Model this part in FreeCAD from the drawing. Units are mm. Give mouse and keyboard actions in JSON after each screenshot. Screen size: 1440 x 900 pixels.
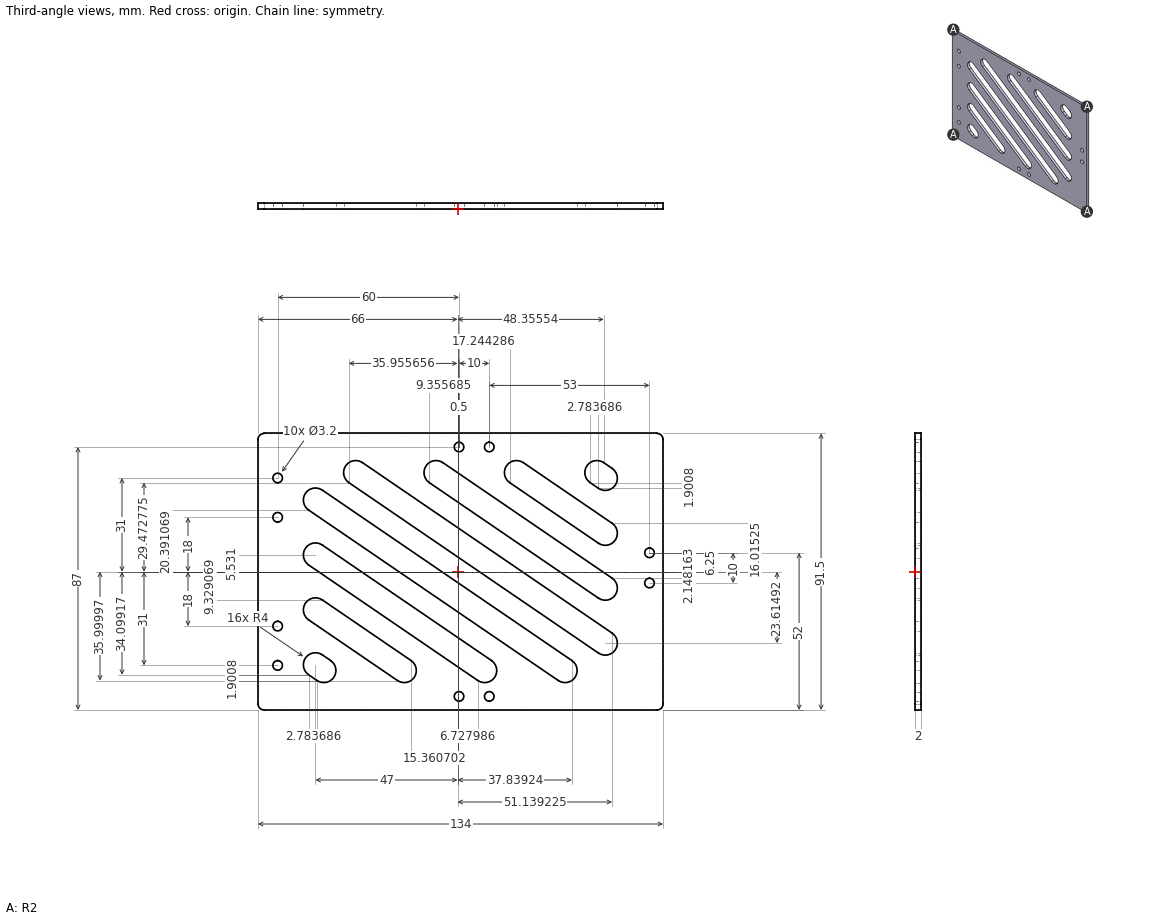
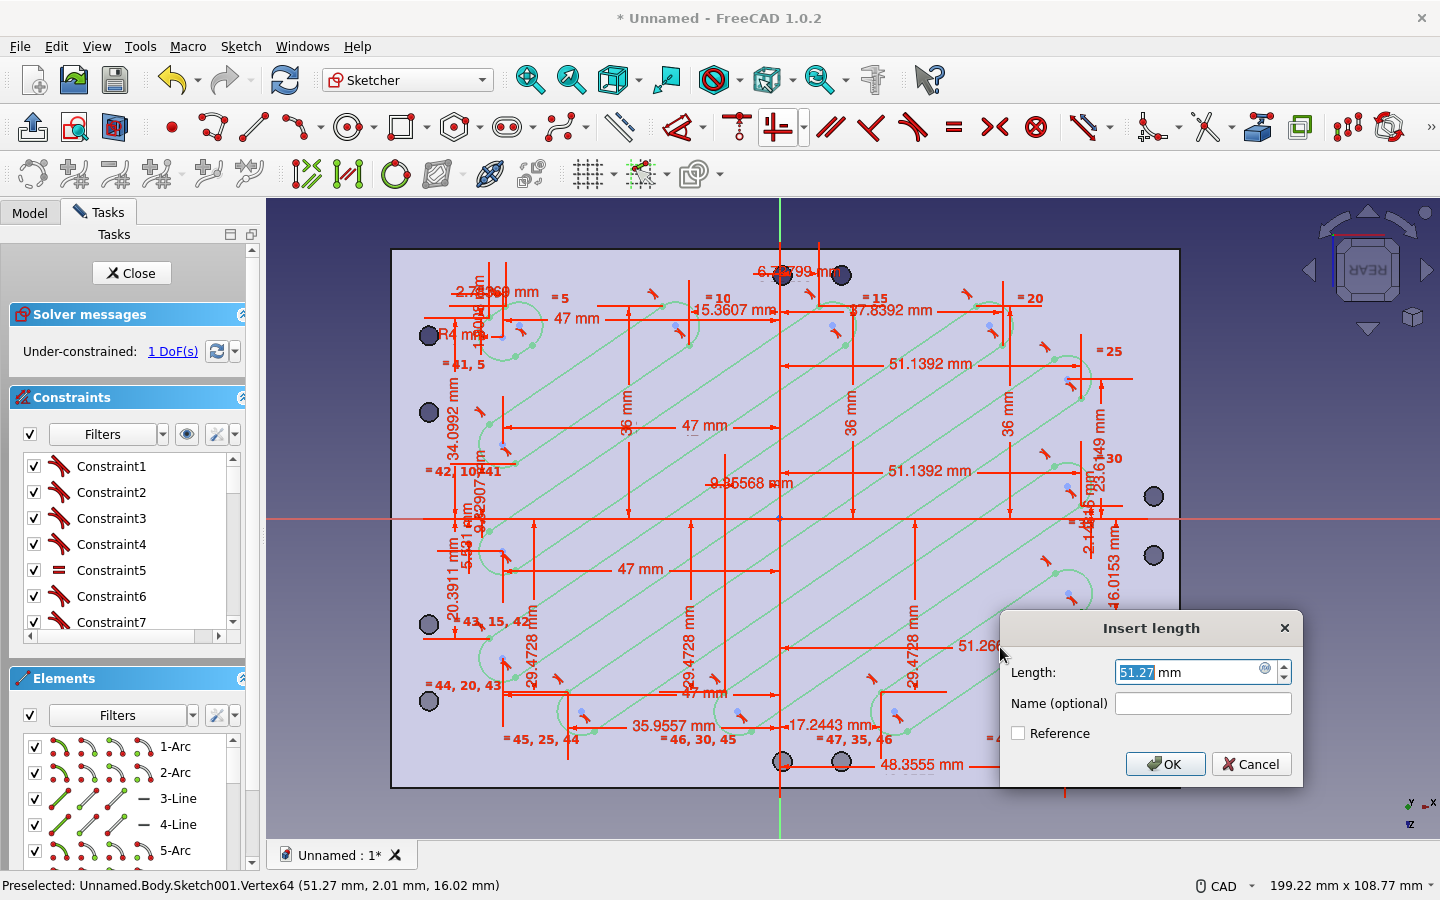
{"action": "type", "text": "51.139225"}
{"action": "key", "text": "Return"}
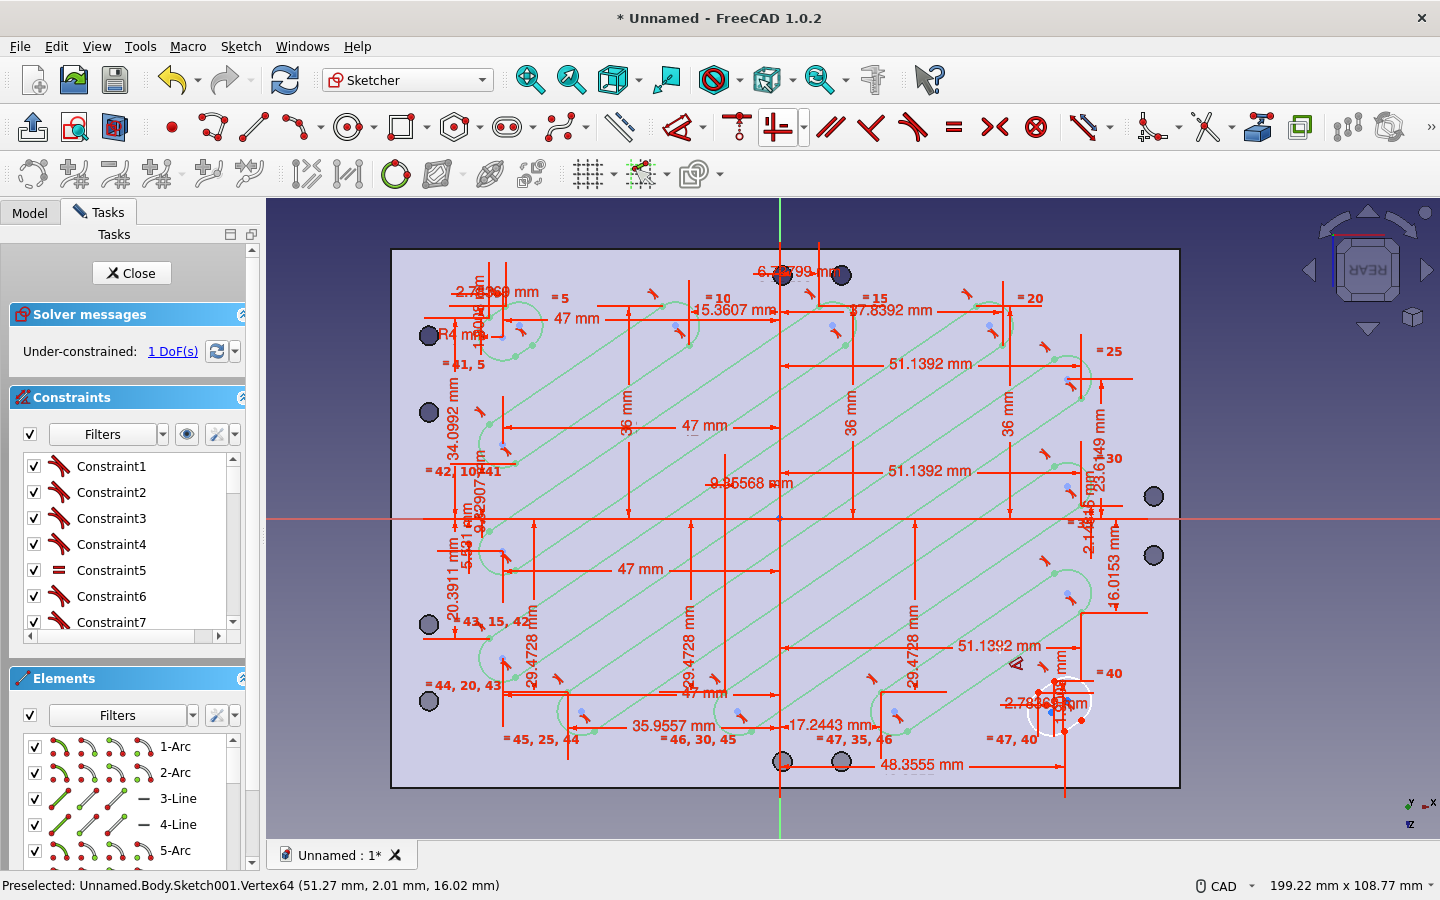
{"action": "left_click", "coordinate": [1038, 693]}
{"action": "left_click", "coordinate": [1072, 646]}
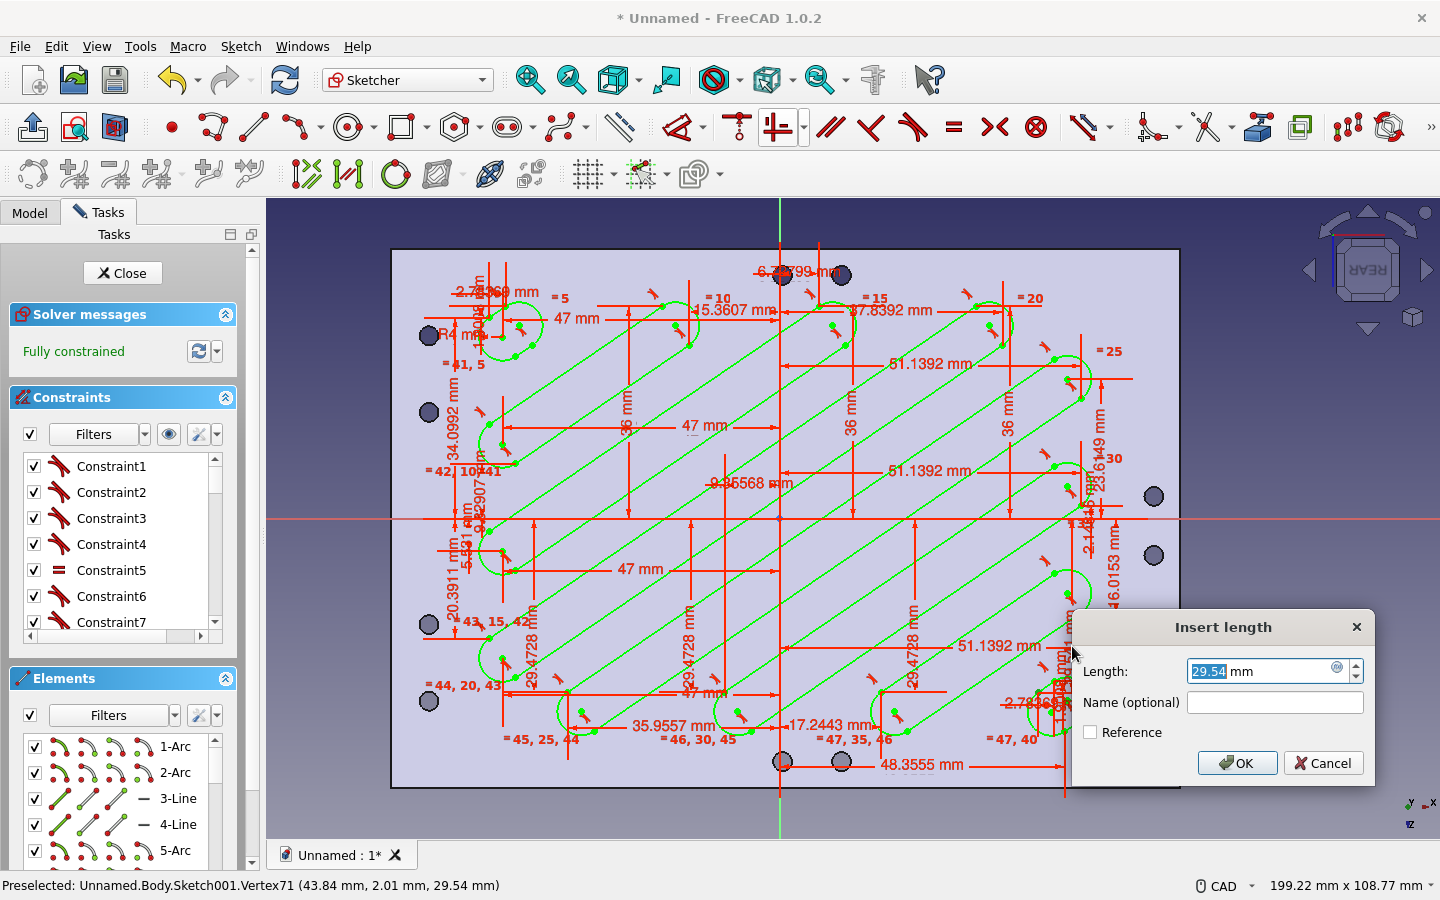
{"action": "type", "text": "29.472775"}
{"action": "key", "text": "Return"}
{"action": "key", "text": "Escape"}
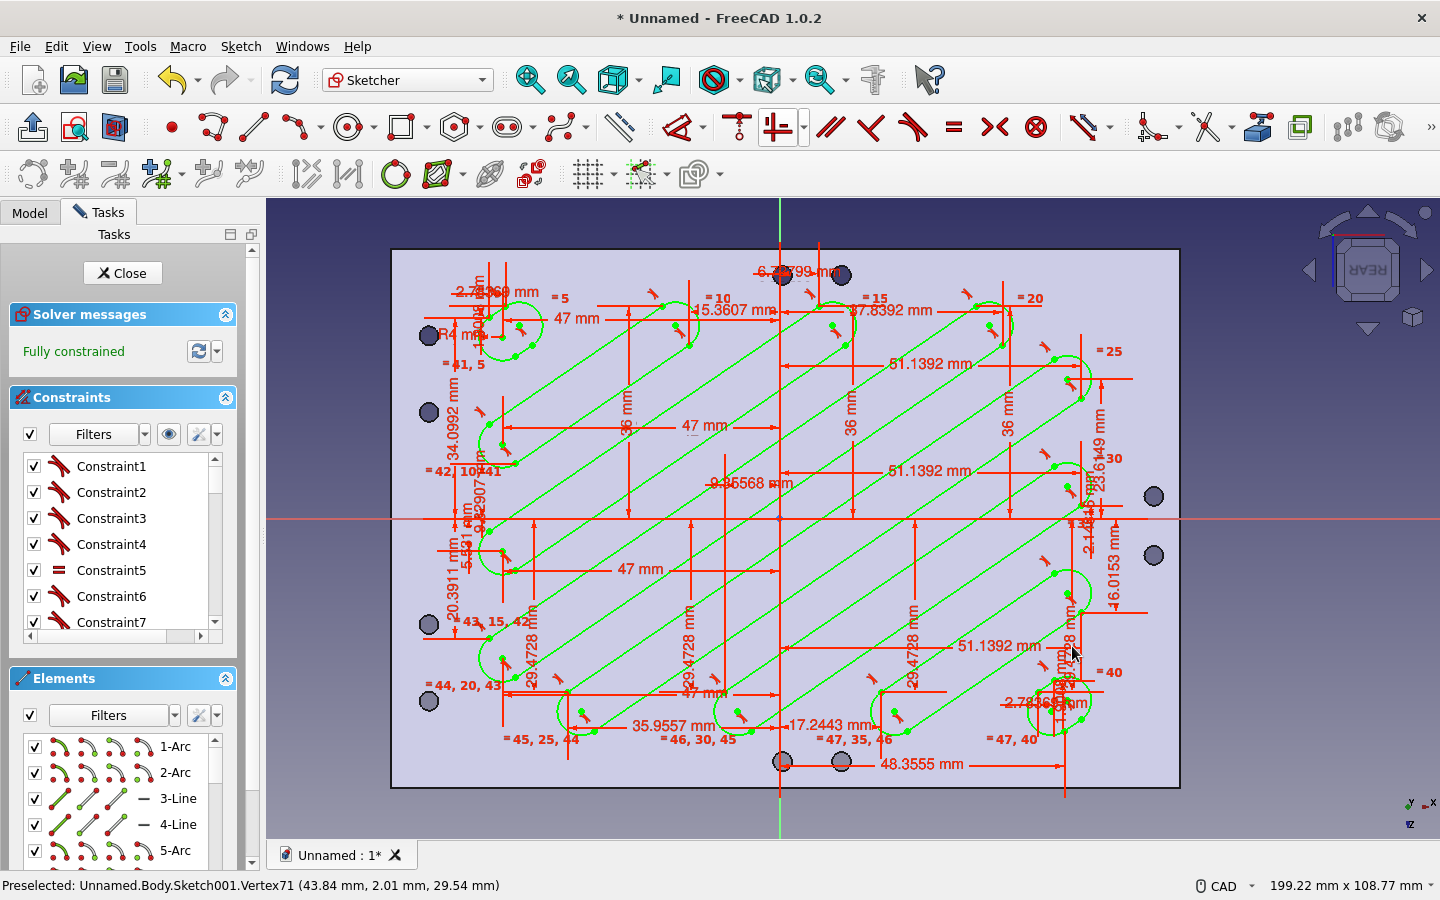
{"action": "left_click", "coordinate": [123, 273]}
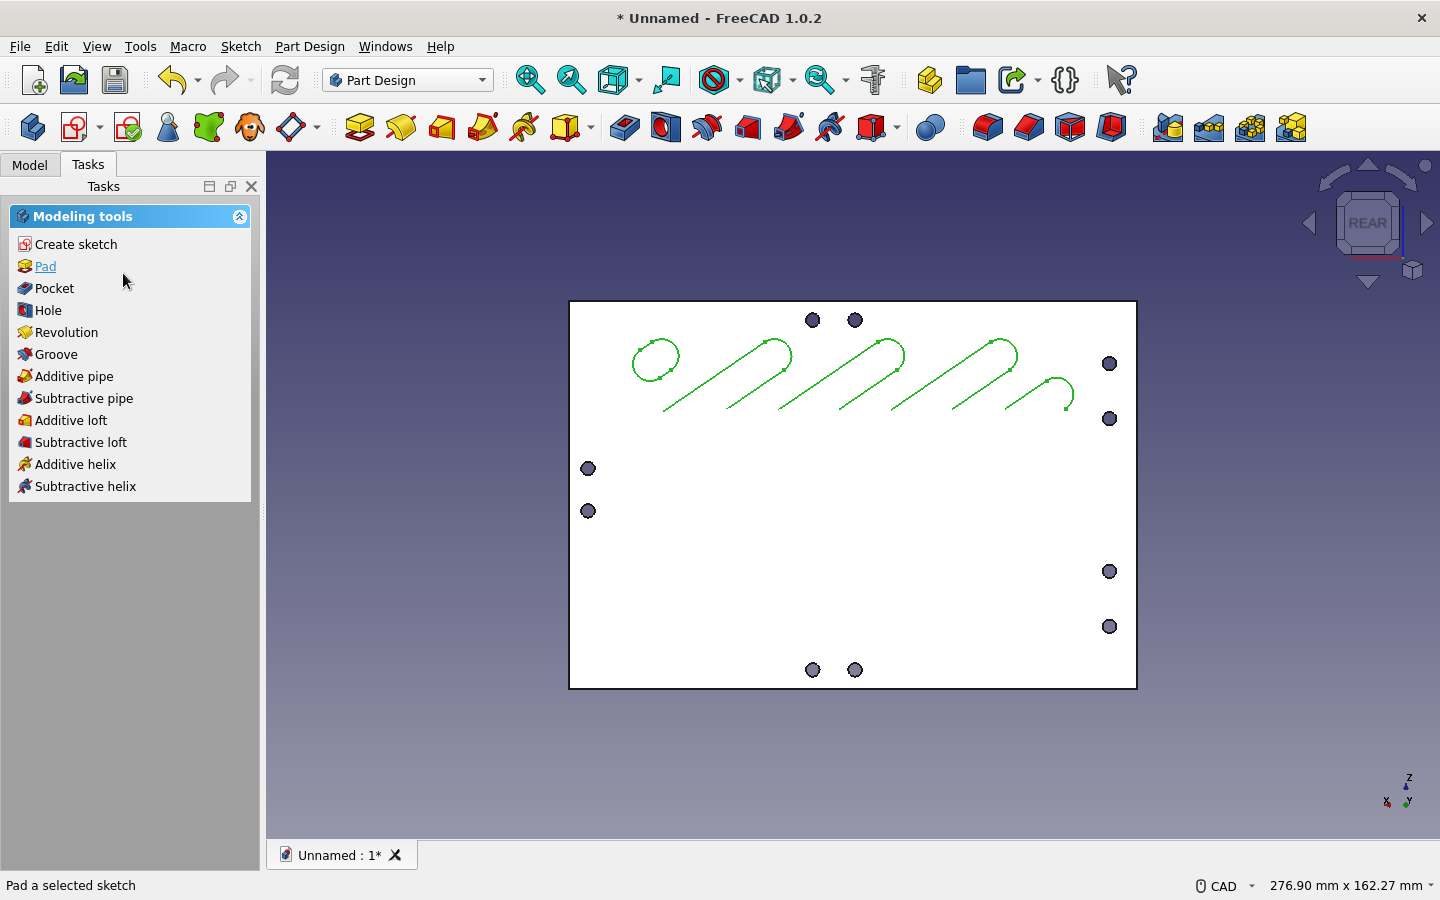
{"action": "left_click", "coordinate": [625, 128]}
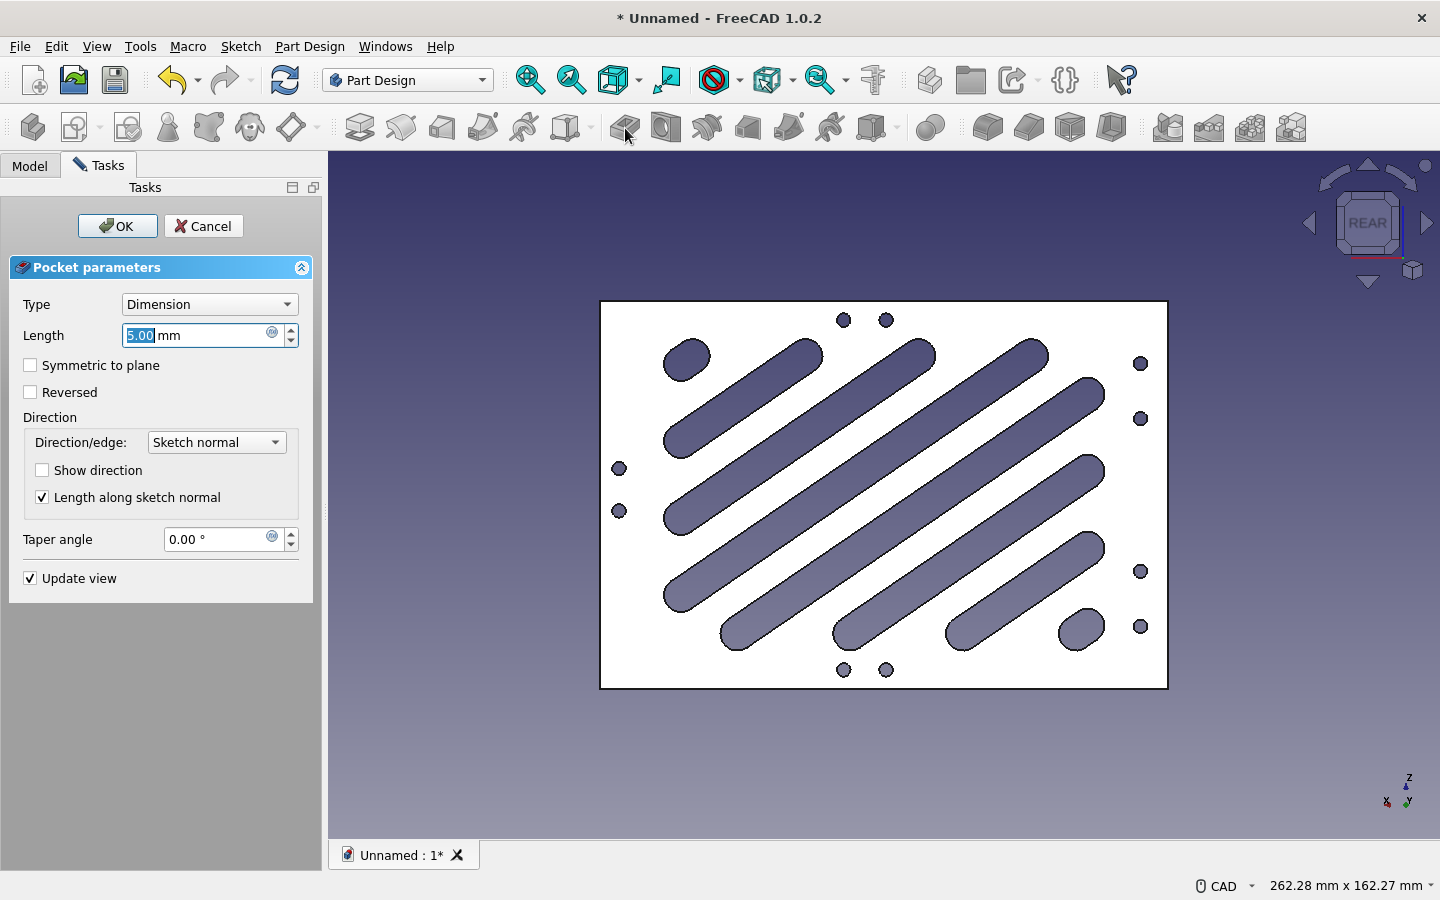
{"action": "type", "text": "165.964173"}
{"action": "key", "text": "Tab"}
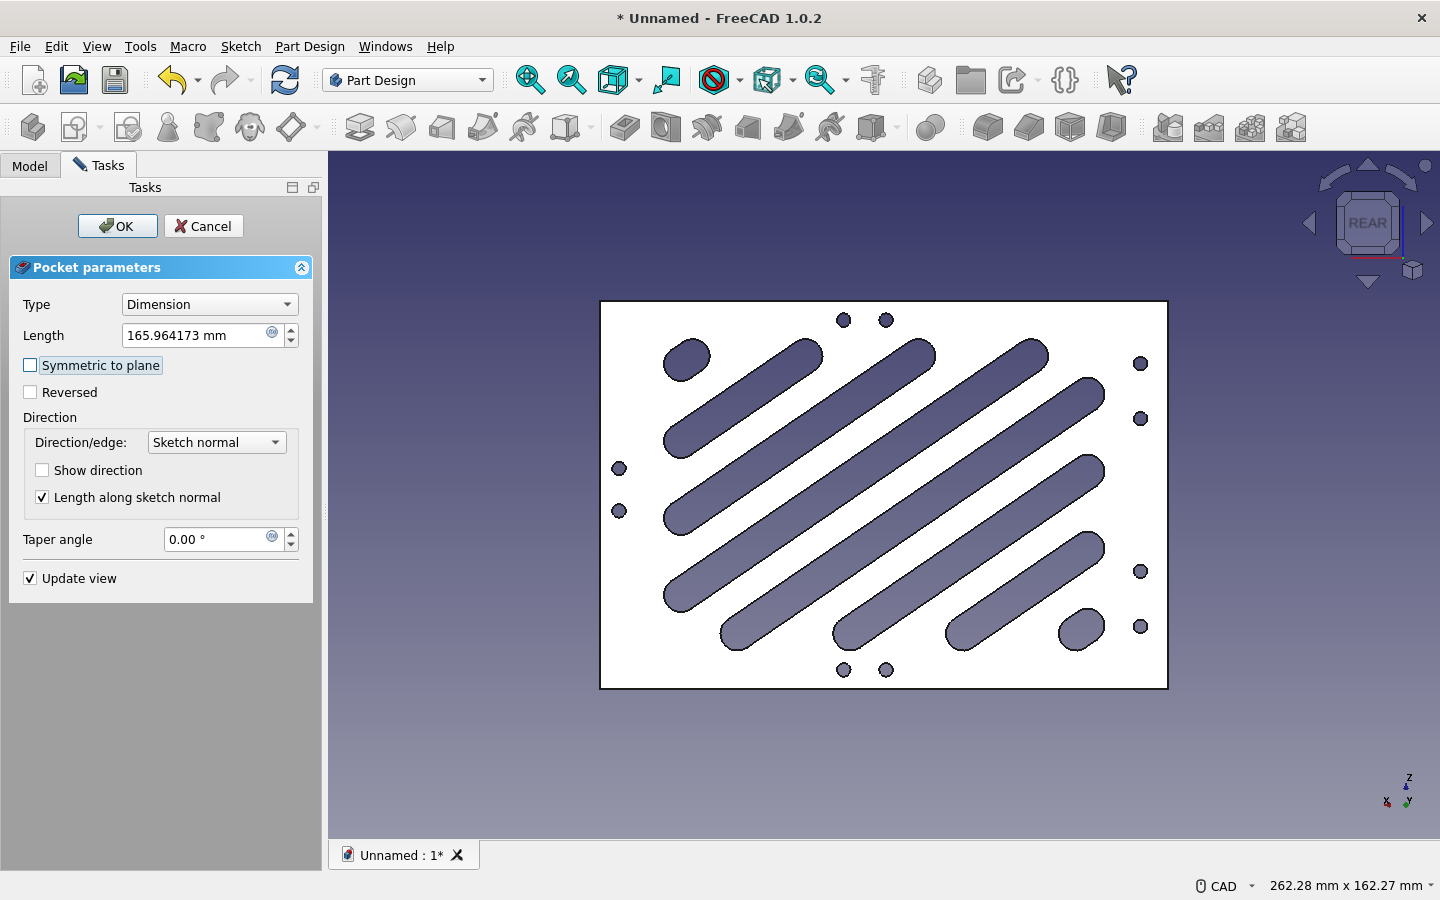
{"action": "left_click", "coordinate": [31, 365]}